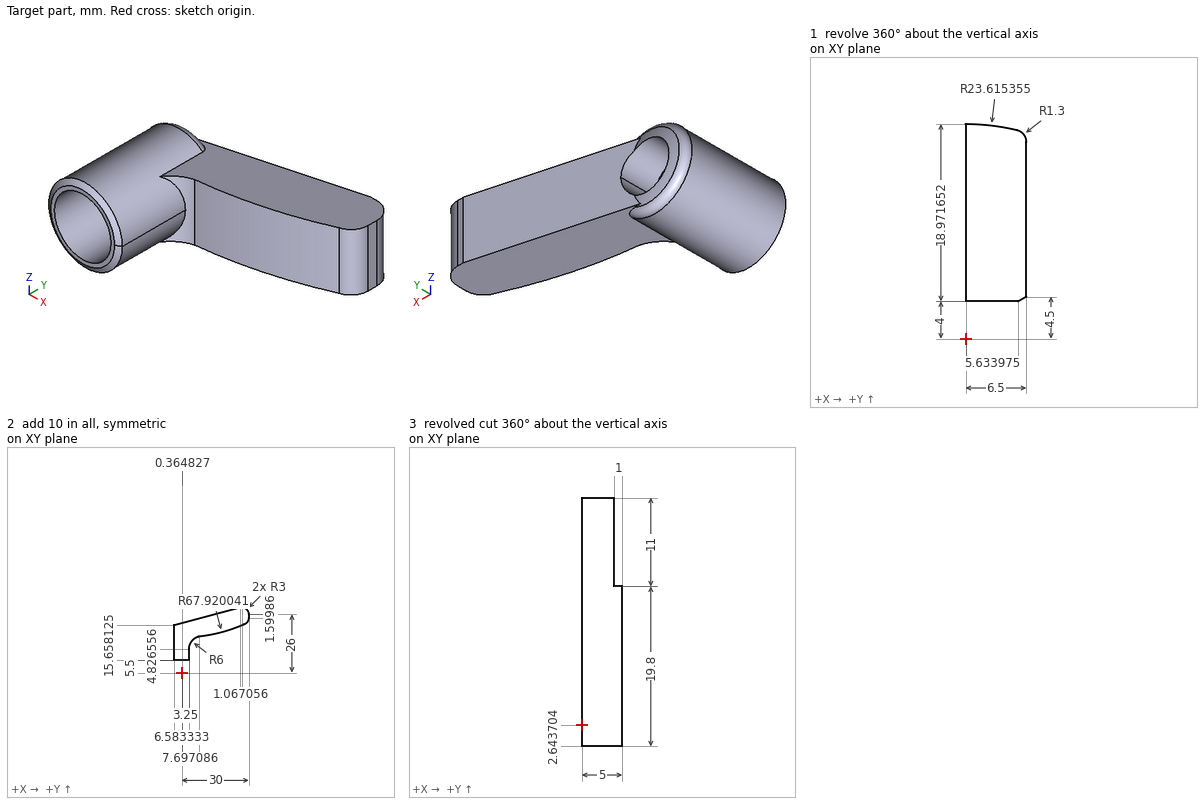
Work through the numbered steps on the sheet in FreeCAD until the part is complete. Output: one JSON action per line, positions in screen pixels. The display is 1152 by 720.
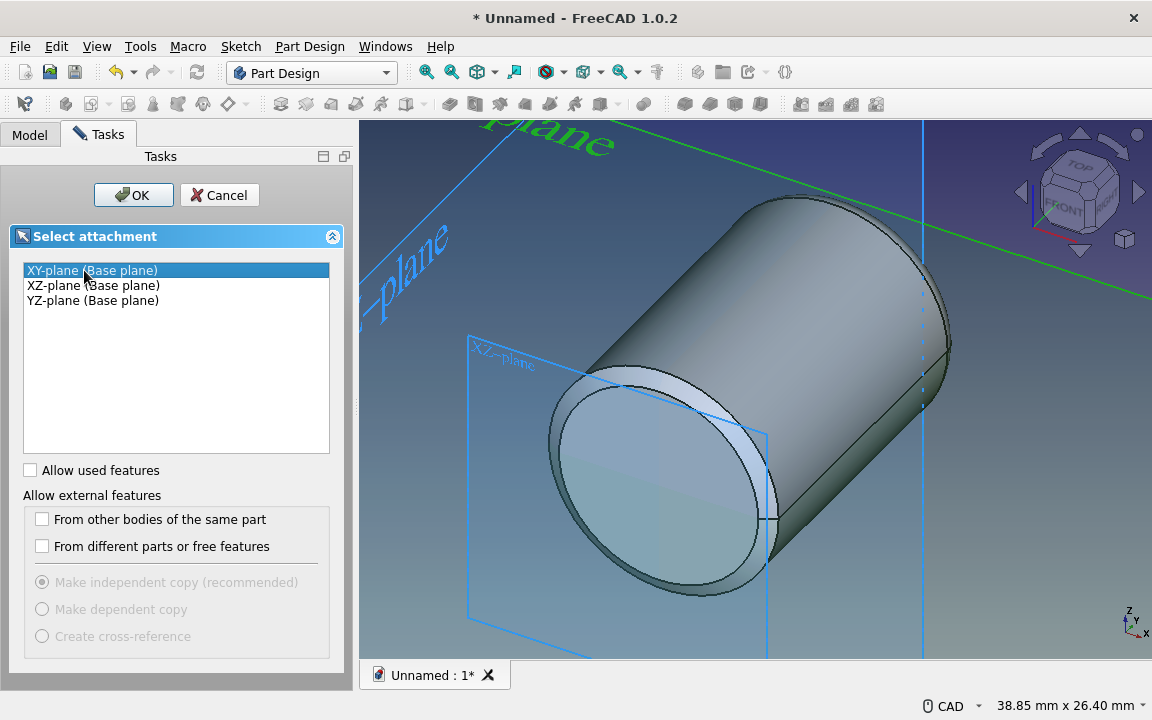
{"action": "left_click", "coordinate": [134, 195]}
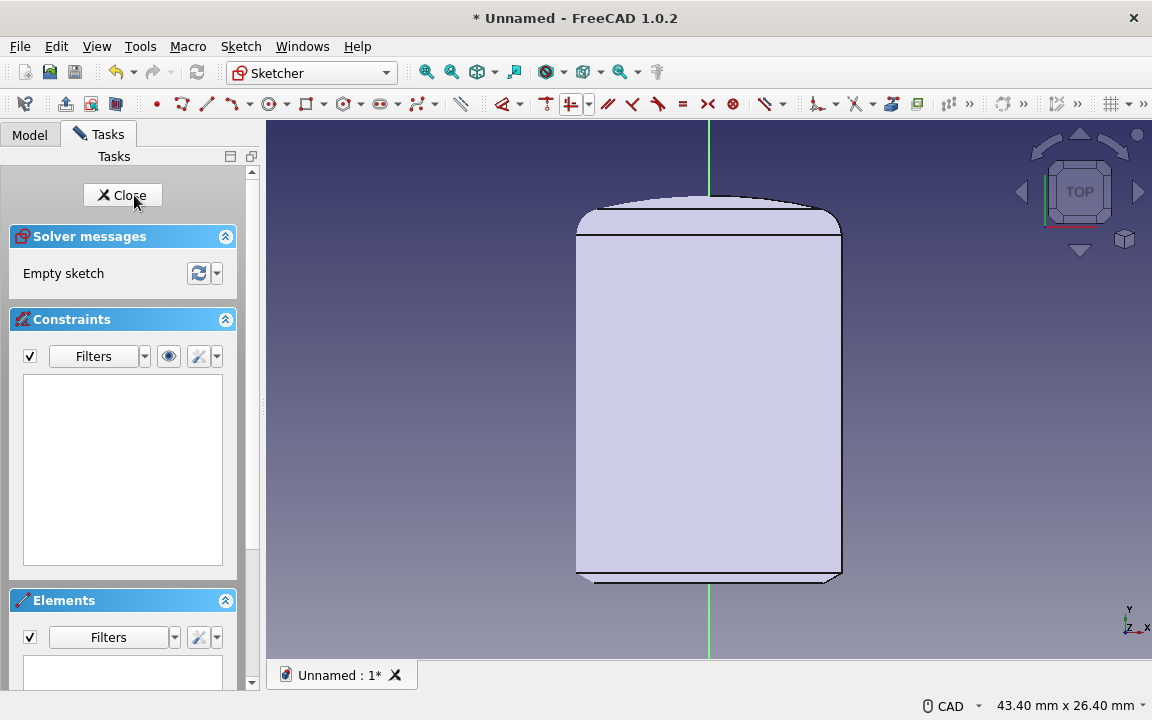
{"action": "key", "text": "q s"}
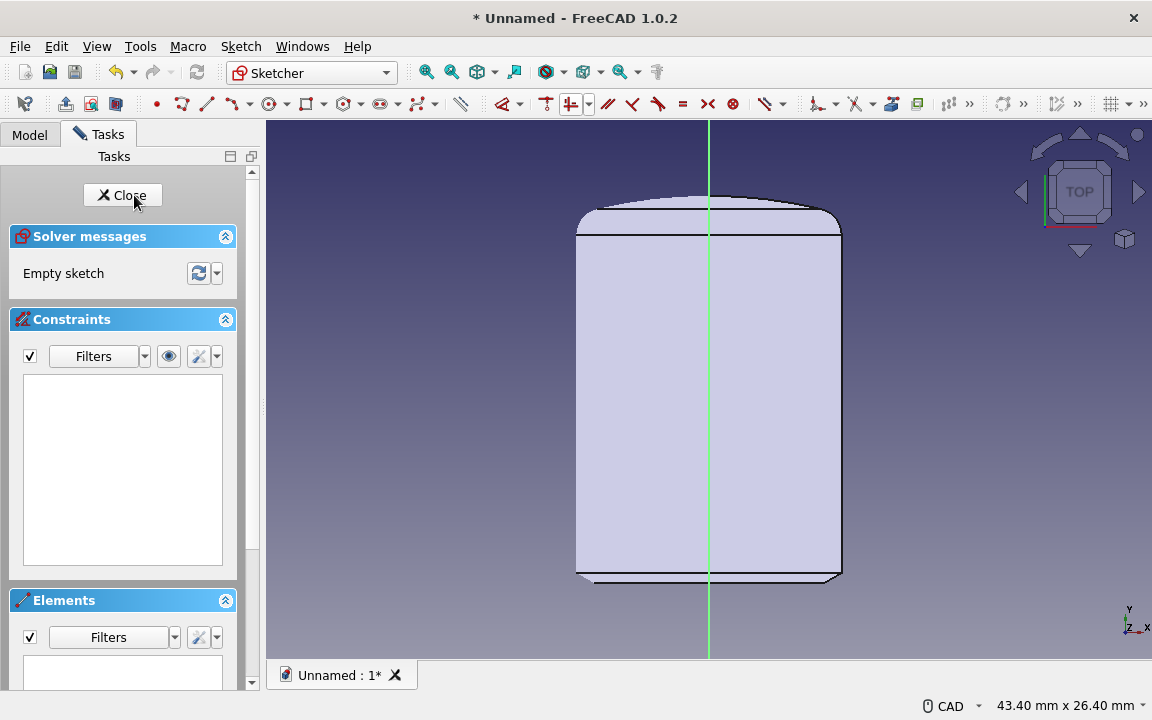
{"action": "scroll", "coordinate": [294, 415], "scroll_direction": "down", "scroll_amount": 3}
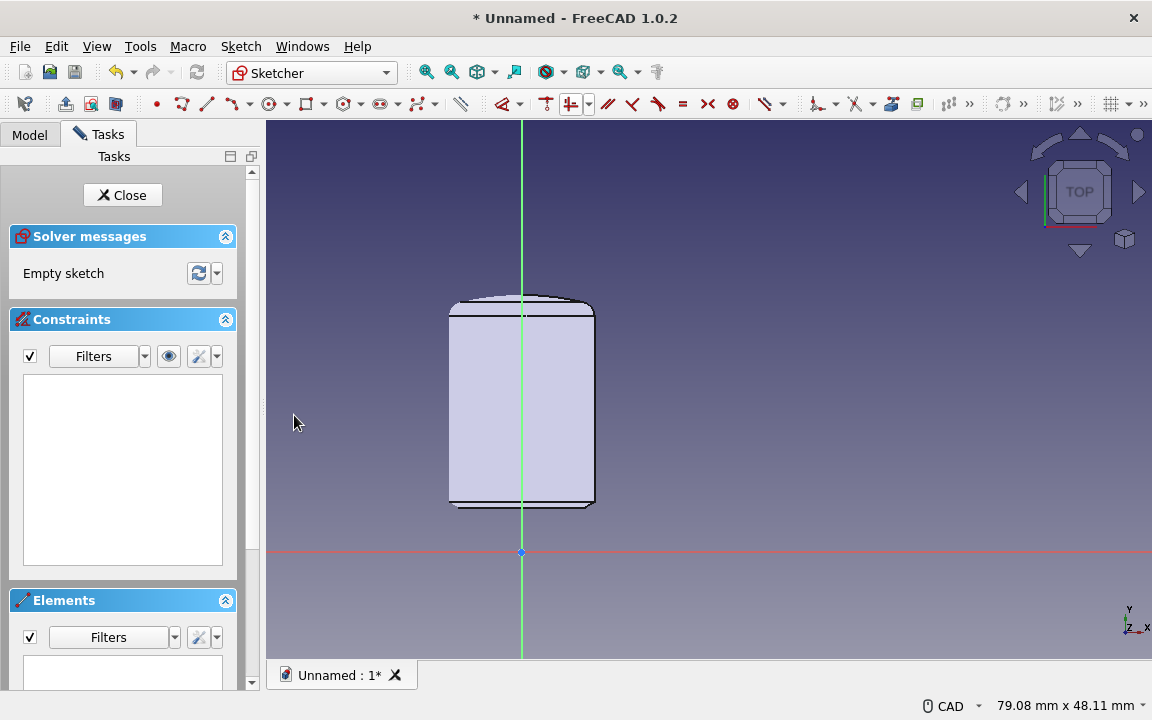
{"action": "key", "text": "g l"}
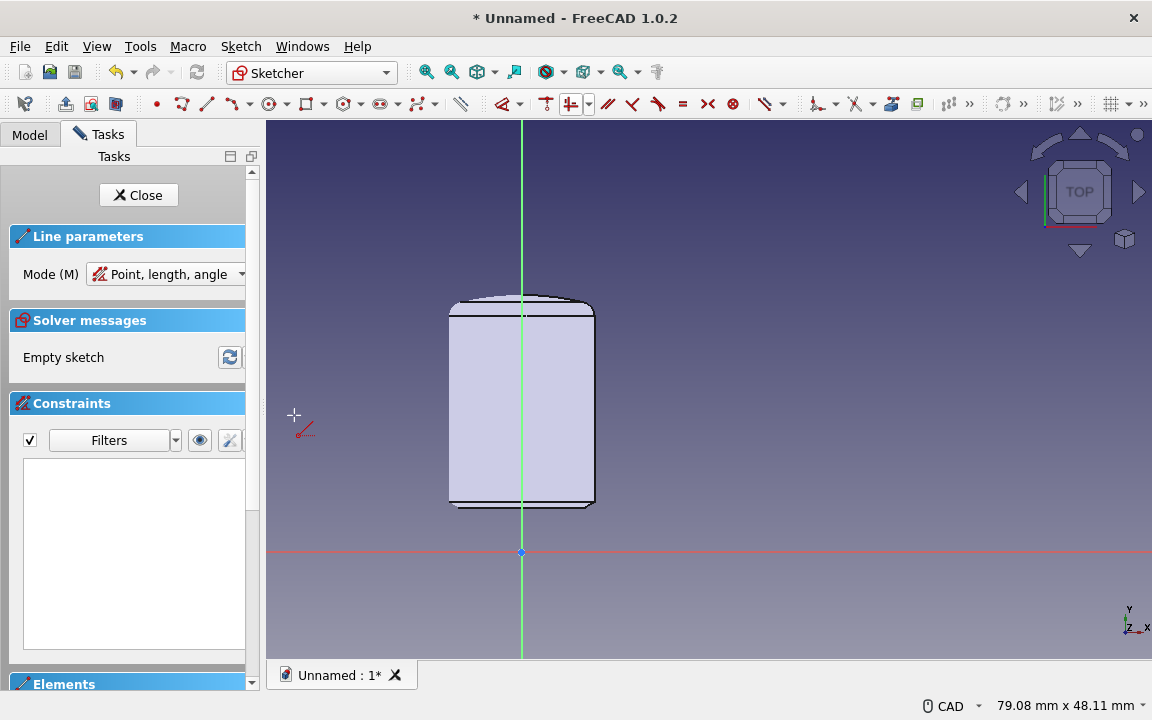
{"action": "left_click", "coordinate": [858, 279]}
{"action": "left_click", "coordinate": [858, 261]}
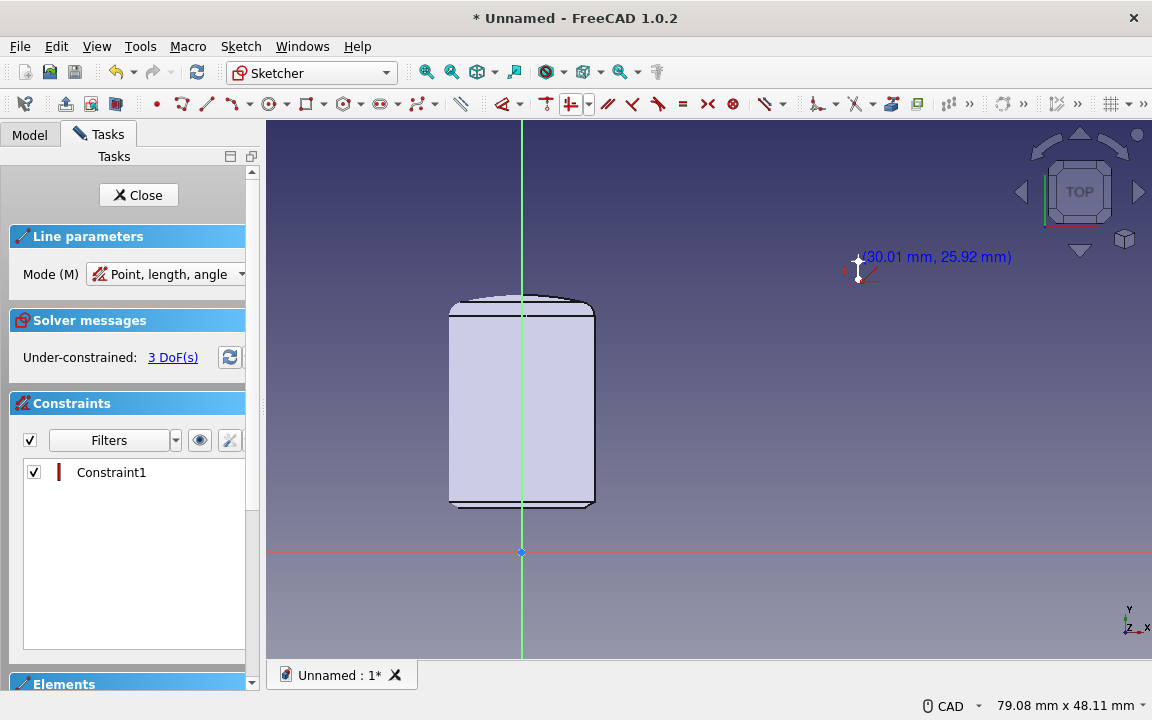
{"action": "key", "text": "g m"}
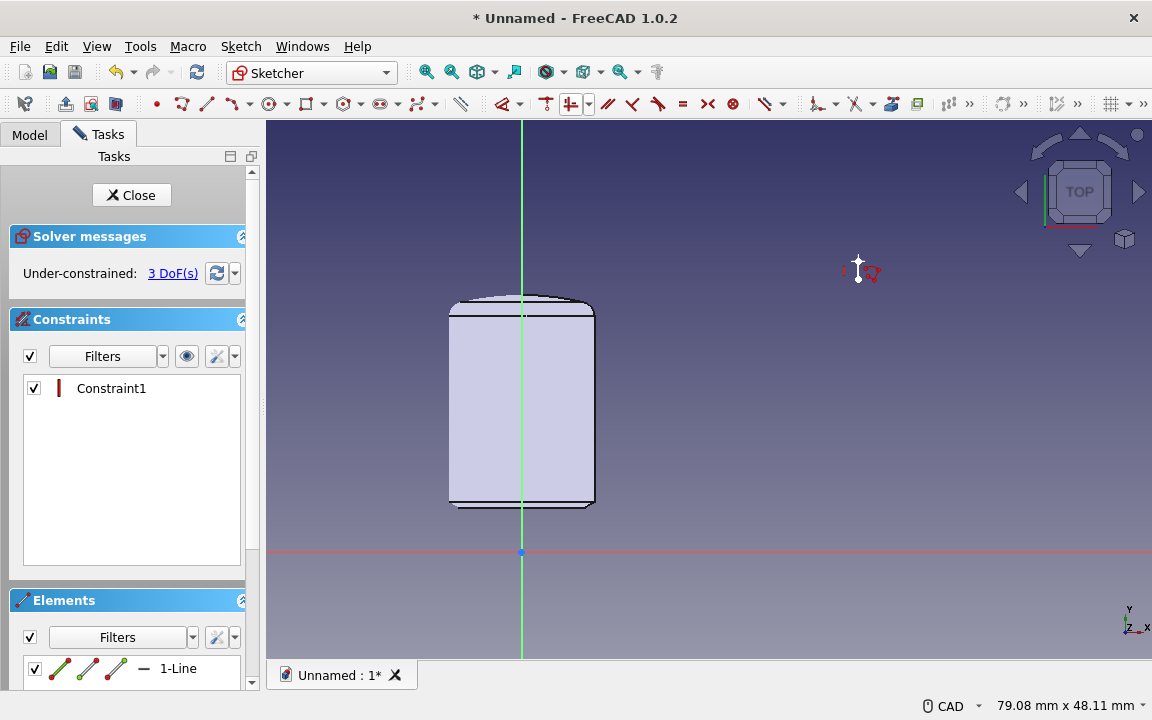
{"action": "left_click", "coordinate": [824, 227]}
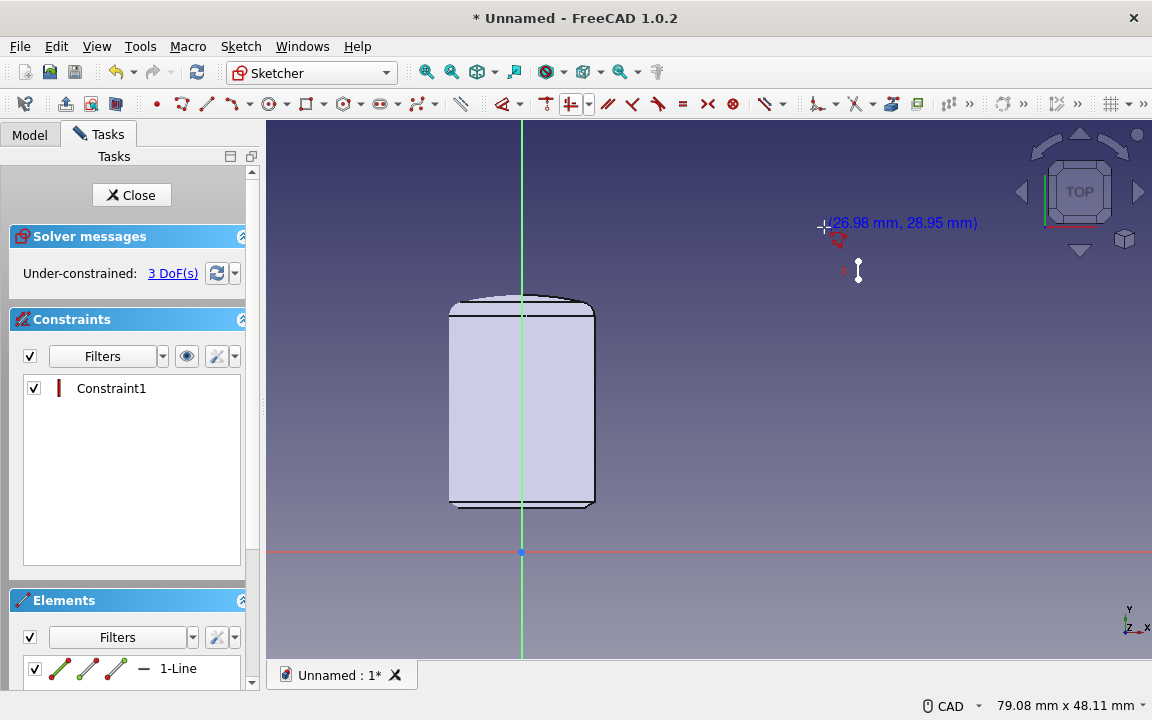
{"action": "scroll", "coordinate": [812, 227], "scroll_direction": "up", "scroll_amount": 2}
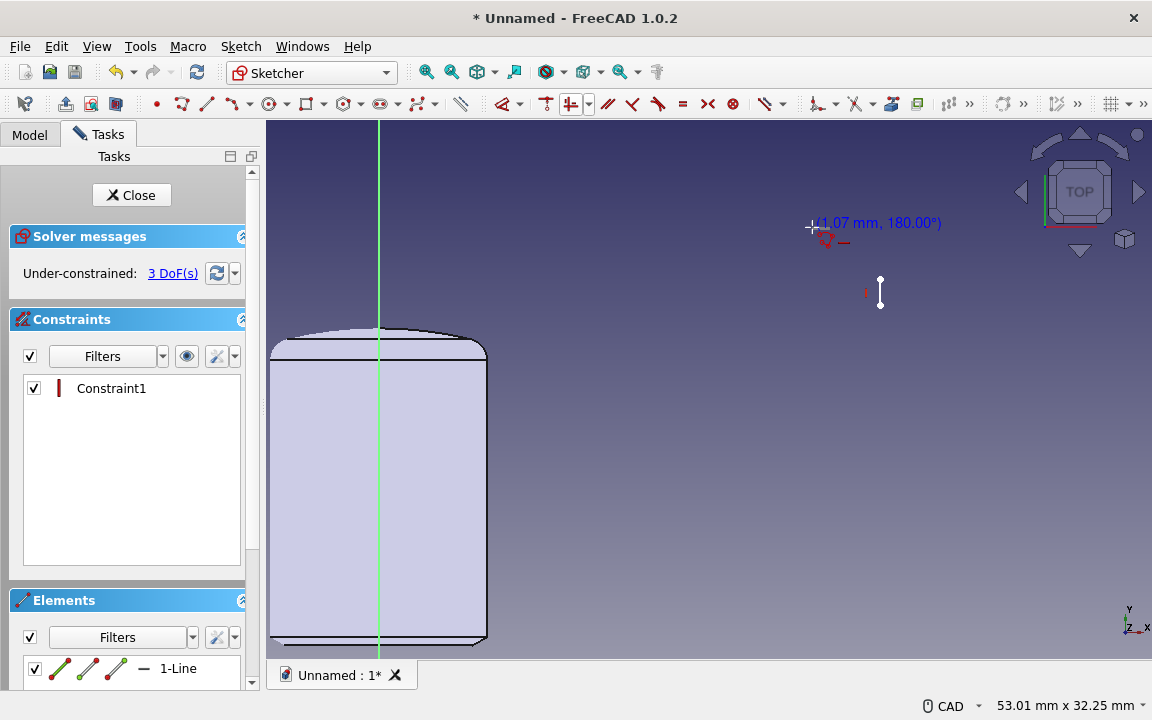
{"action": "left_click", "coordinate": [812, 227]}
{"action": "left_click", "coordinate": [323, 359]}
{"action": "left_click", "coordinate": [323, 620]}
{"action": "left_click", "coordinate": [433, 620]}
{"action": "left_click", "coordinate": [433, 540]}
{"action": "right_click", "coordinate": [433, 540]}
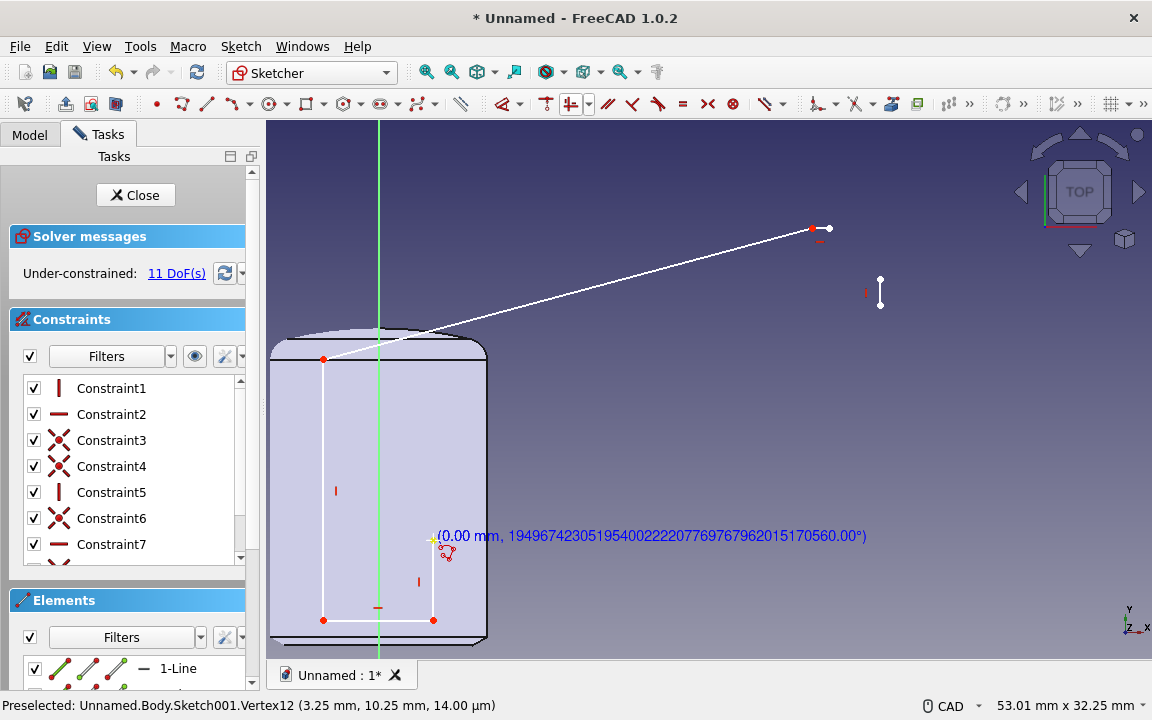
{"action": "key", "text": "g 3 a"}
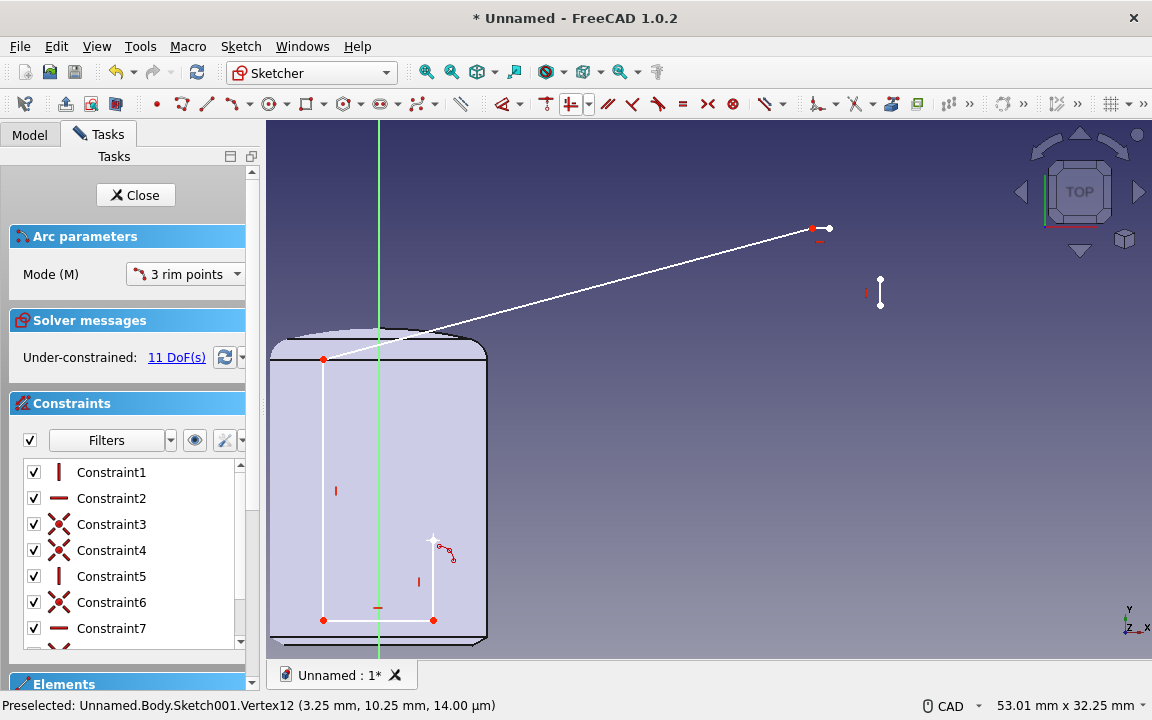
{"action": "left_click", "coordinate": [880, 279]}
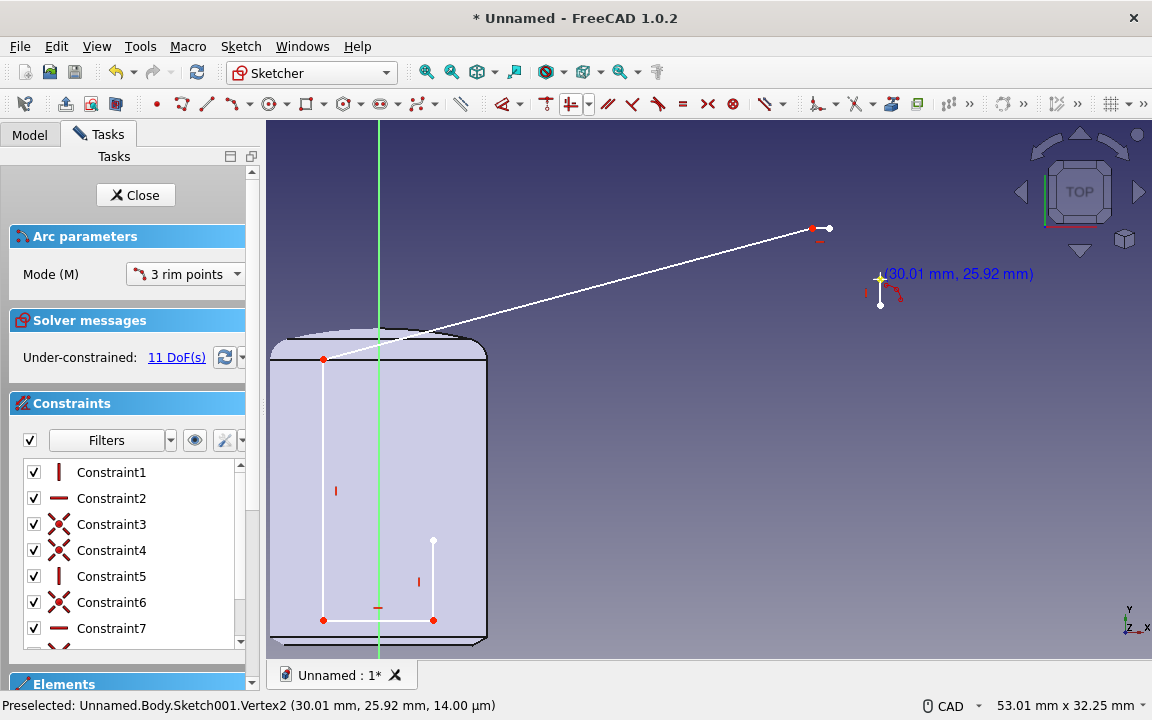
{"action": "scroll", "coordinate": [830, 228], "scroll_direction": "up", "scroll_amount": 3}